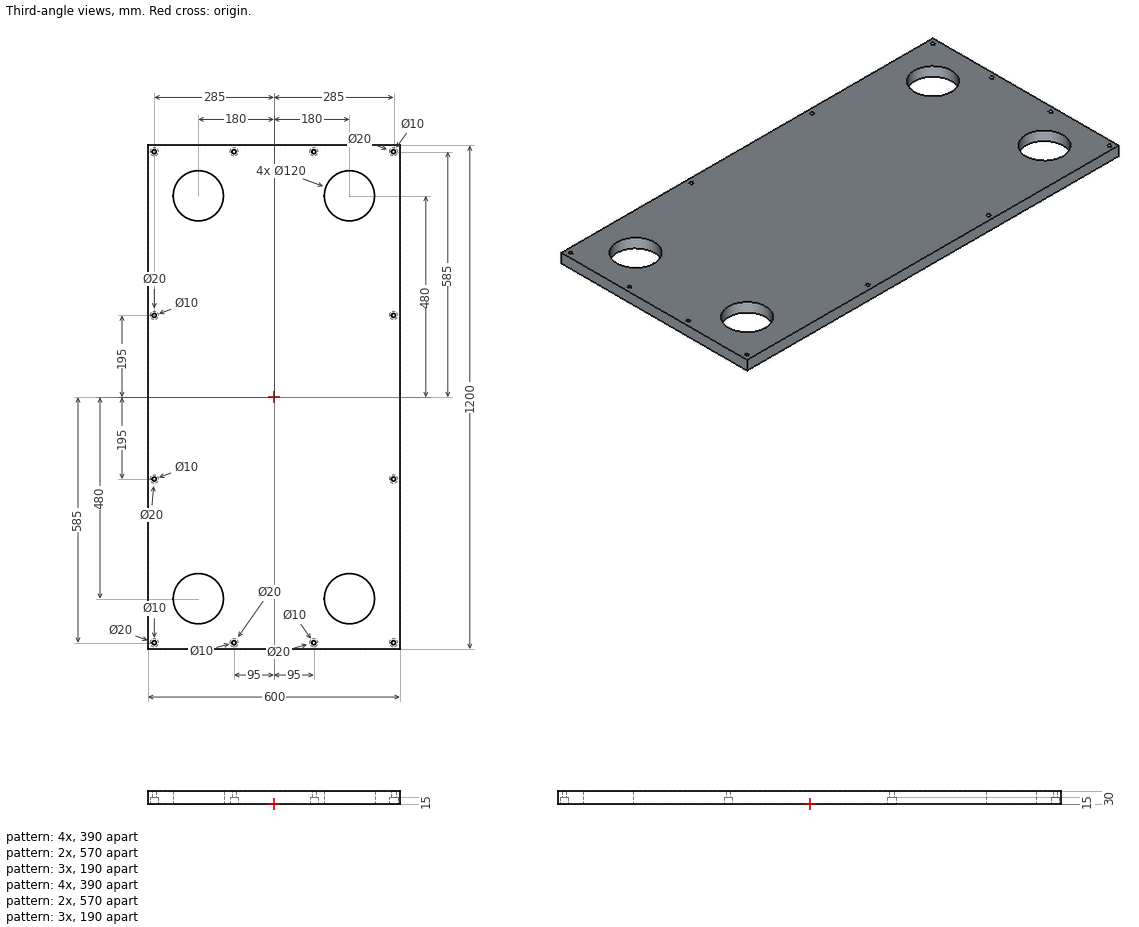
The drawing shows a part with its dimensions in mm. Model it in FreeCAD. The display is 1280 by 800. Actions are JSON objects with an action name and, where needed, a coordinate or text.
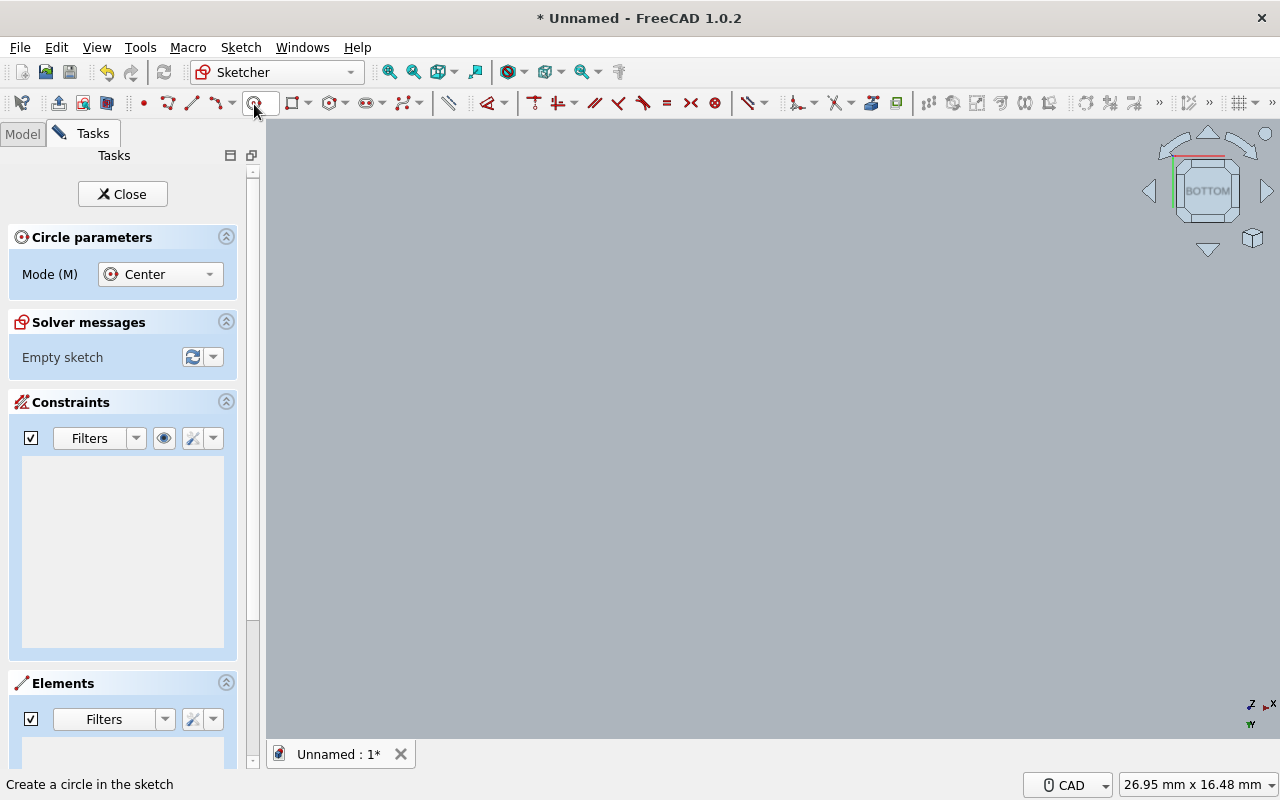
{"action": "left_click", "coordinate": [703, 428]}
{"action": "mouse_move", "coordinate": [836, 295]}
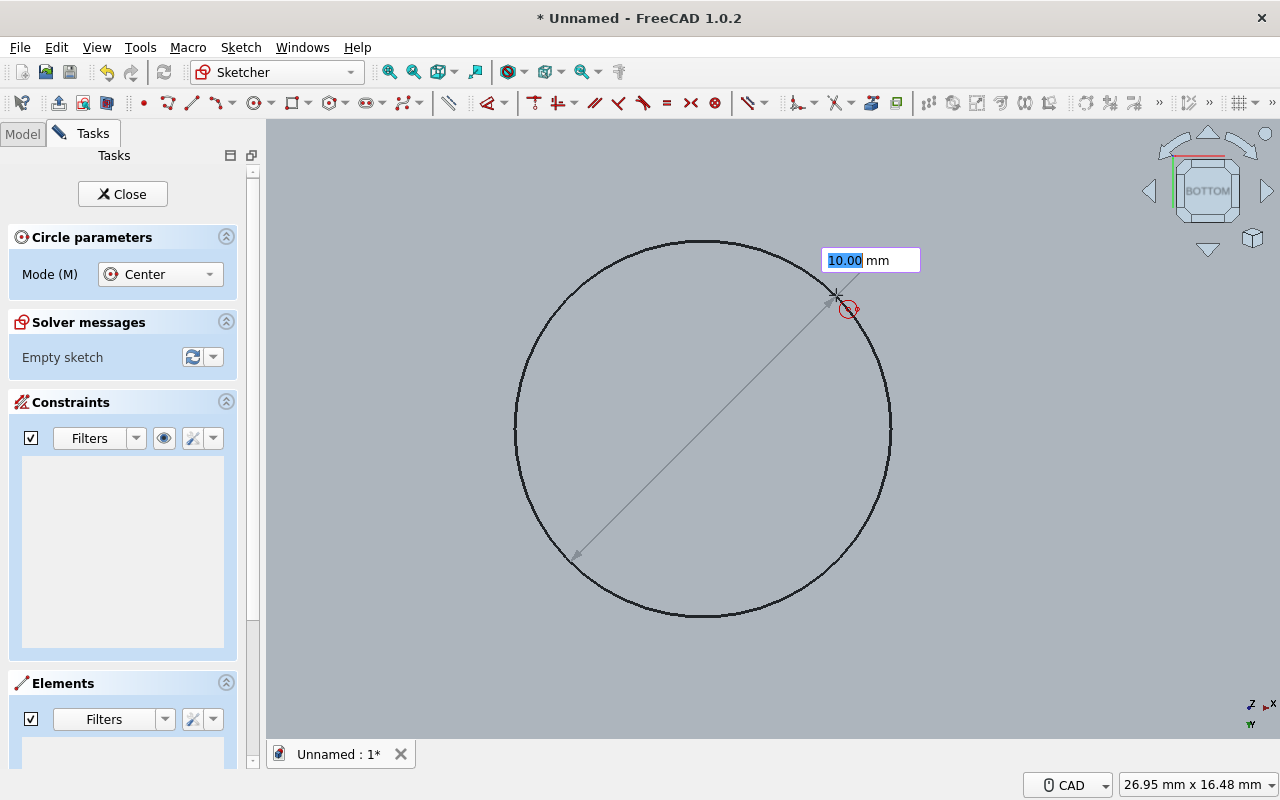
{"action": "type", "text": "10"}
{"action": "key", "text": "Return"}
{"action": "key", "text": "Escape"}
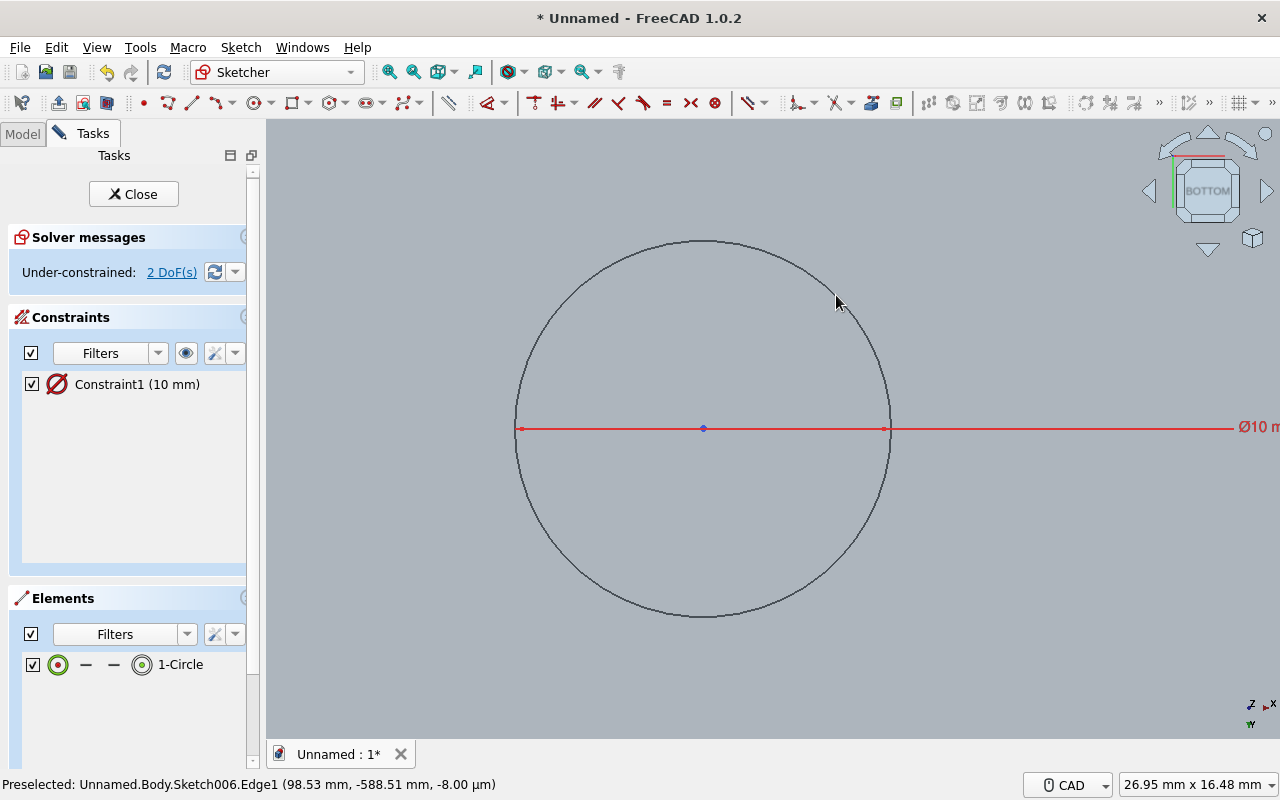
{"action": "left_click", "coordinate": [488, 104]}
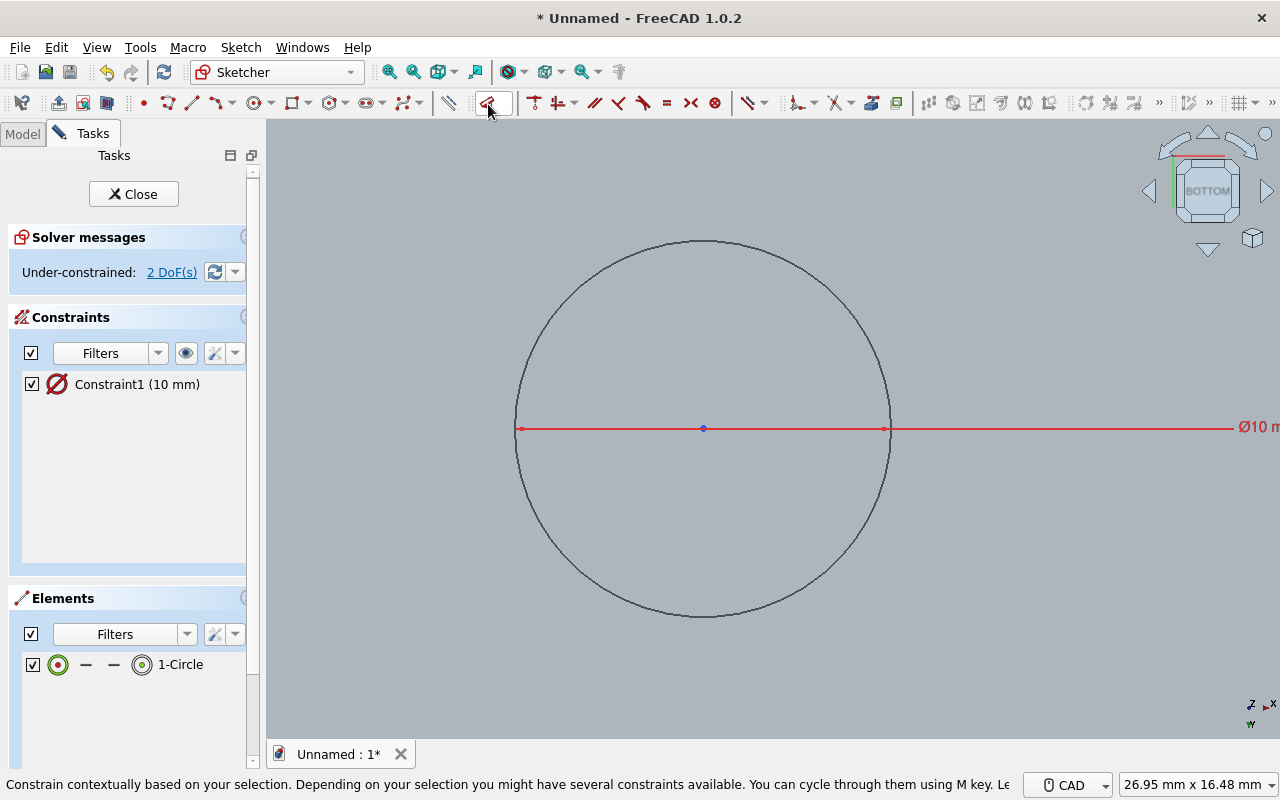
{"action": "left_click", "coordinate": [703, 429]}
{"action": "left_click", "coordinate": [498, 395]}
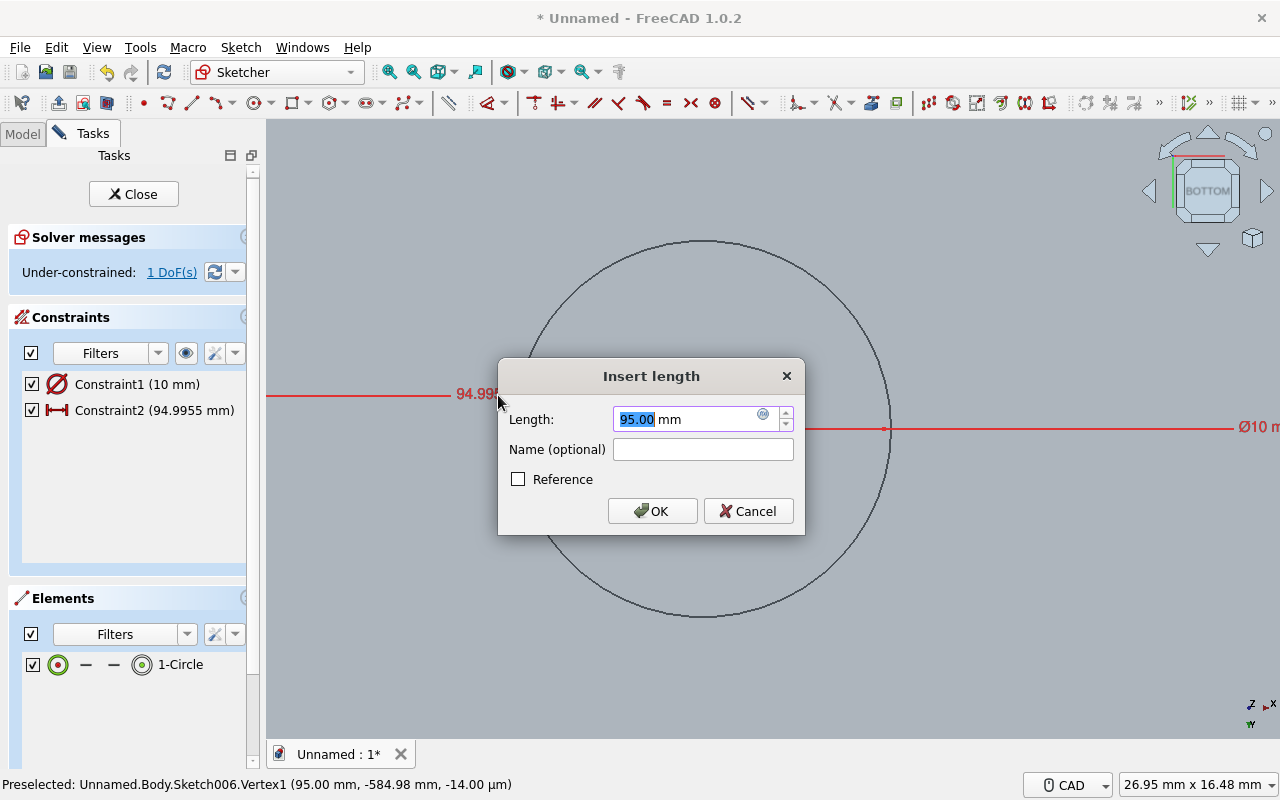
{"action": "type", "text": "95"}
{"action": "key", "text": "Return"}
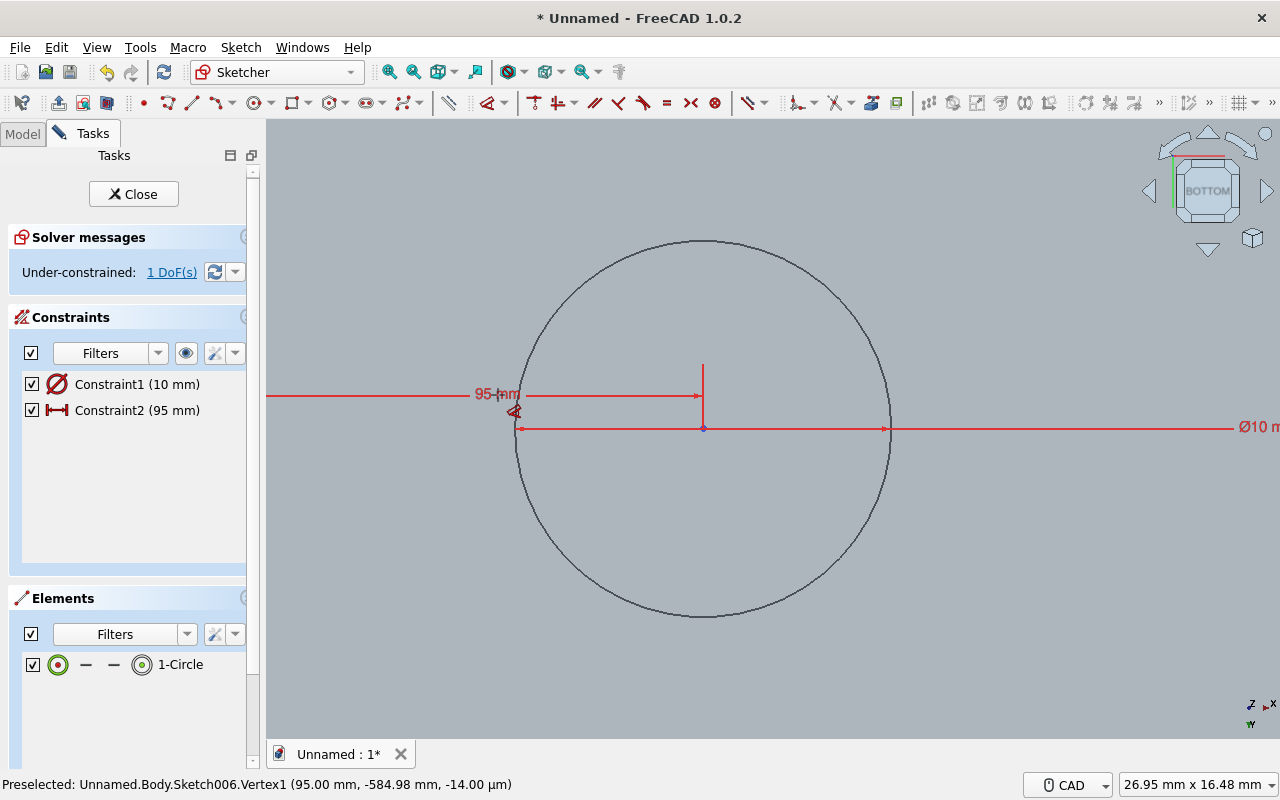
{"action": "left_click", "coordinate": [703, 429]}
{"action": "left_click", "coordinate": [737, 570]}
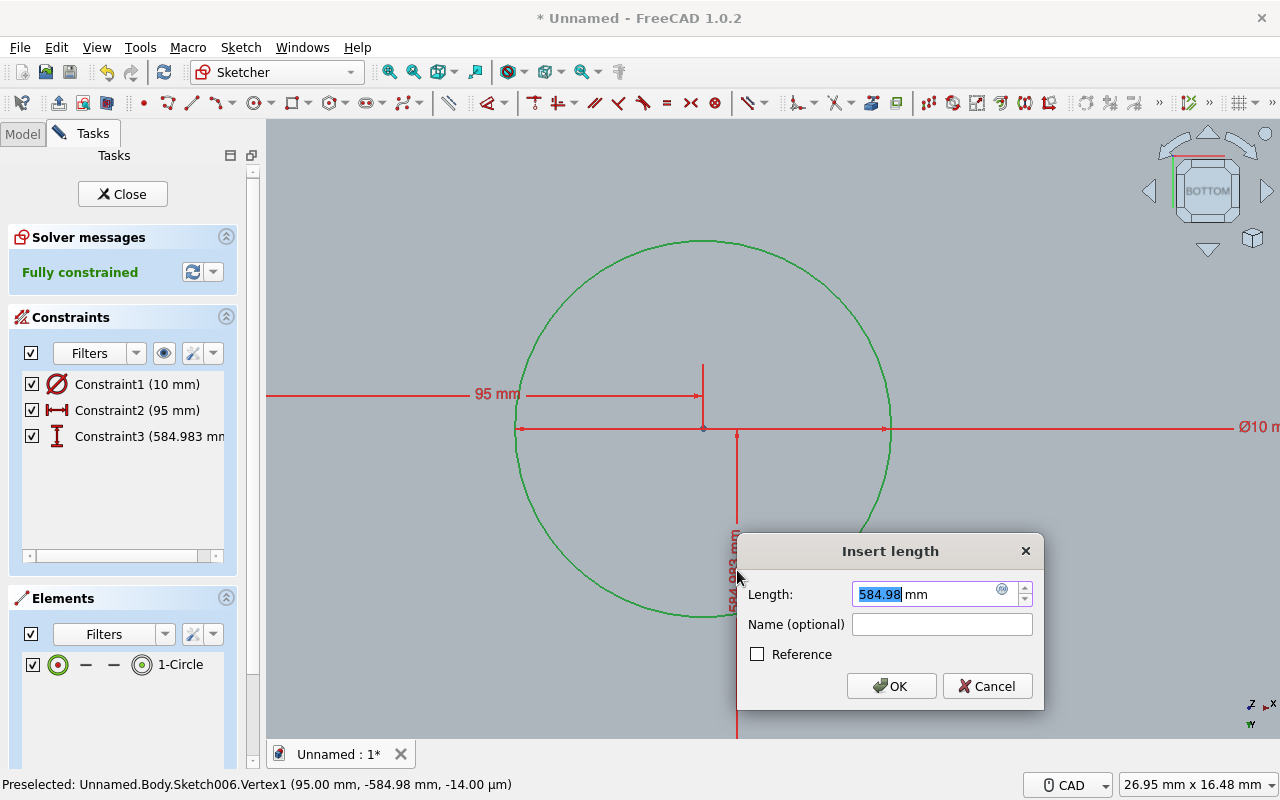
{"action": "type", "text": "585"}
{"action": "key", "text": "Return"}
{"action": "key", "text": "Escape"}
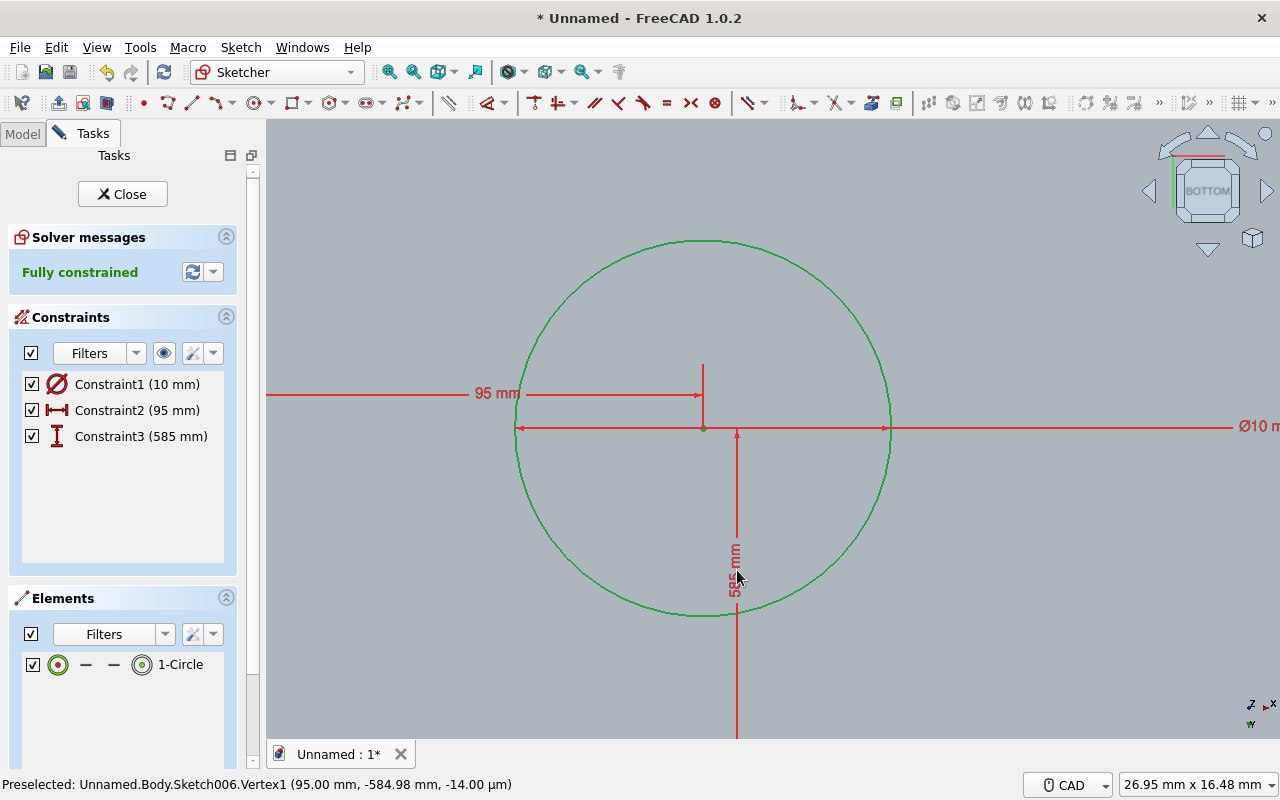
{"action": "left_click", "coordinate": [123, 194]}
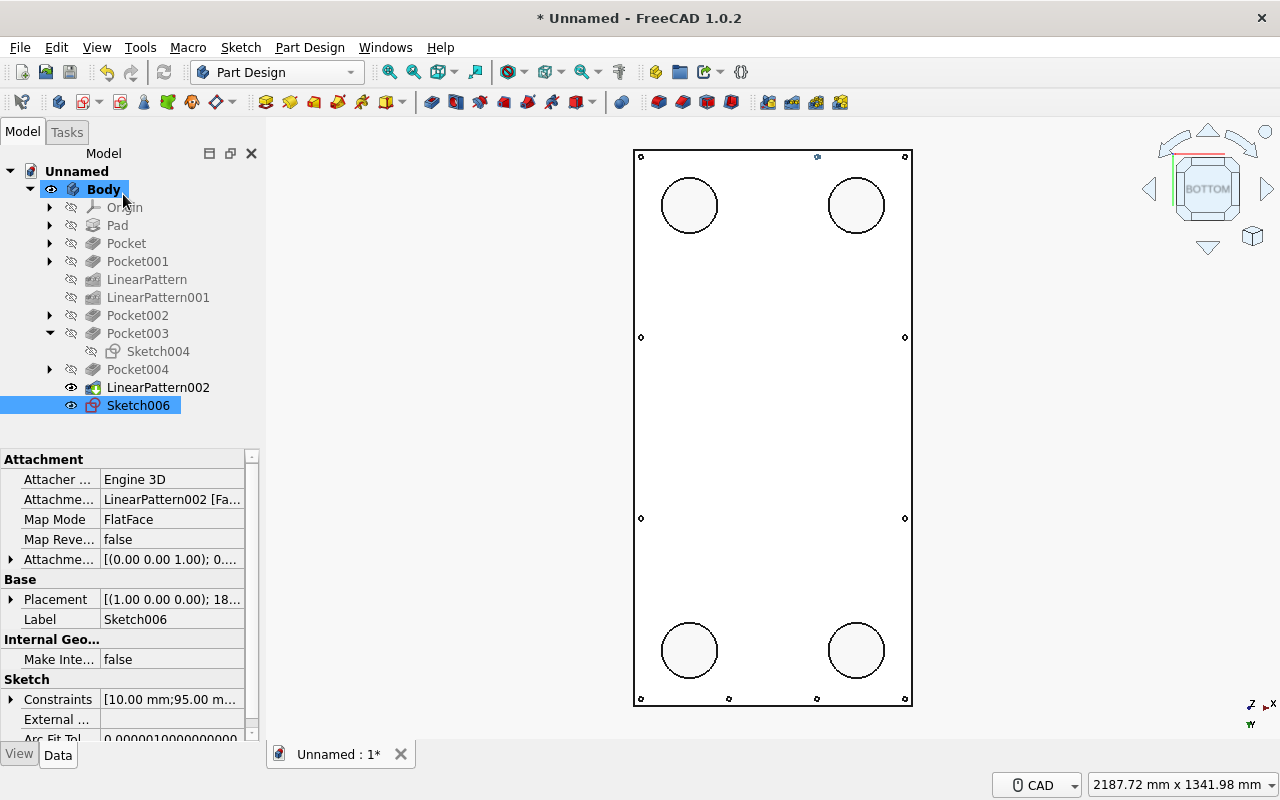
{"action": "left_click", "coordinate": [432, 102]}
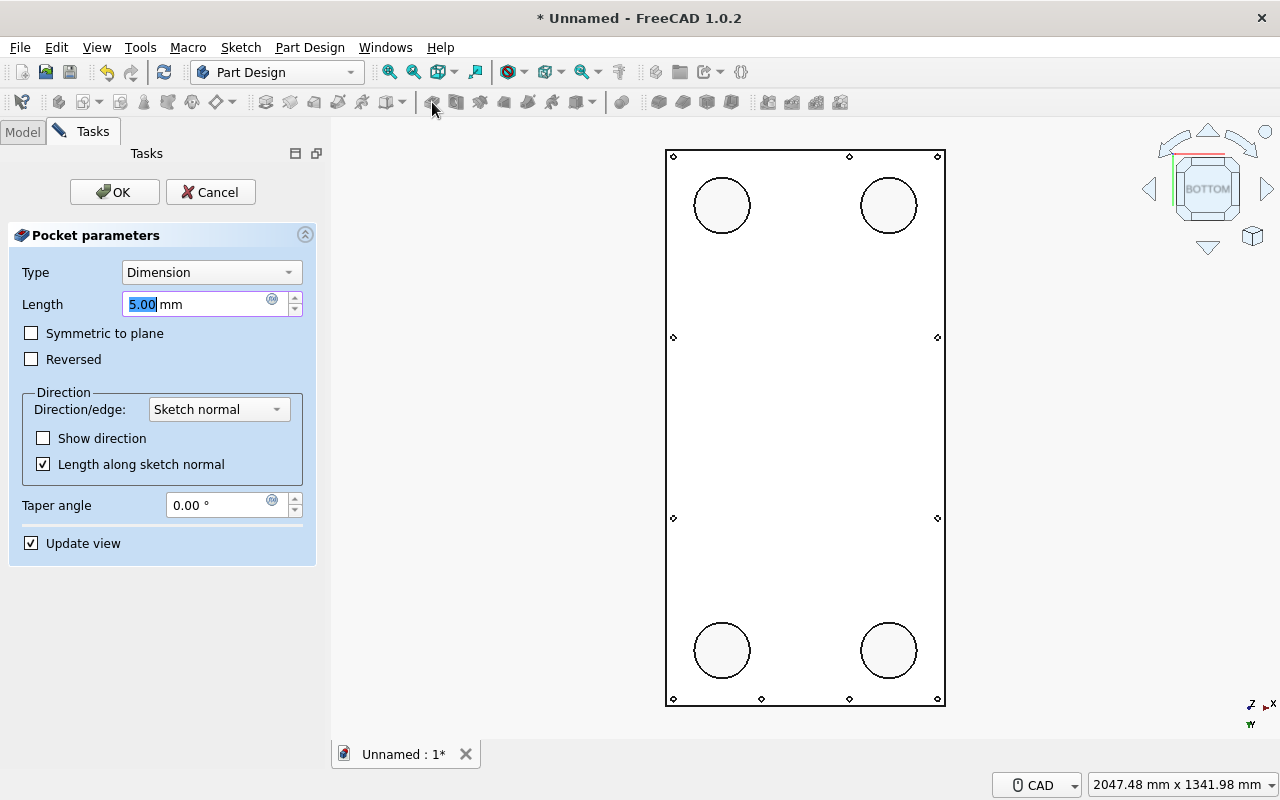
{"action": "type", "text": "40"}
{"action": "key", "text": "Tab"}